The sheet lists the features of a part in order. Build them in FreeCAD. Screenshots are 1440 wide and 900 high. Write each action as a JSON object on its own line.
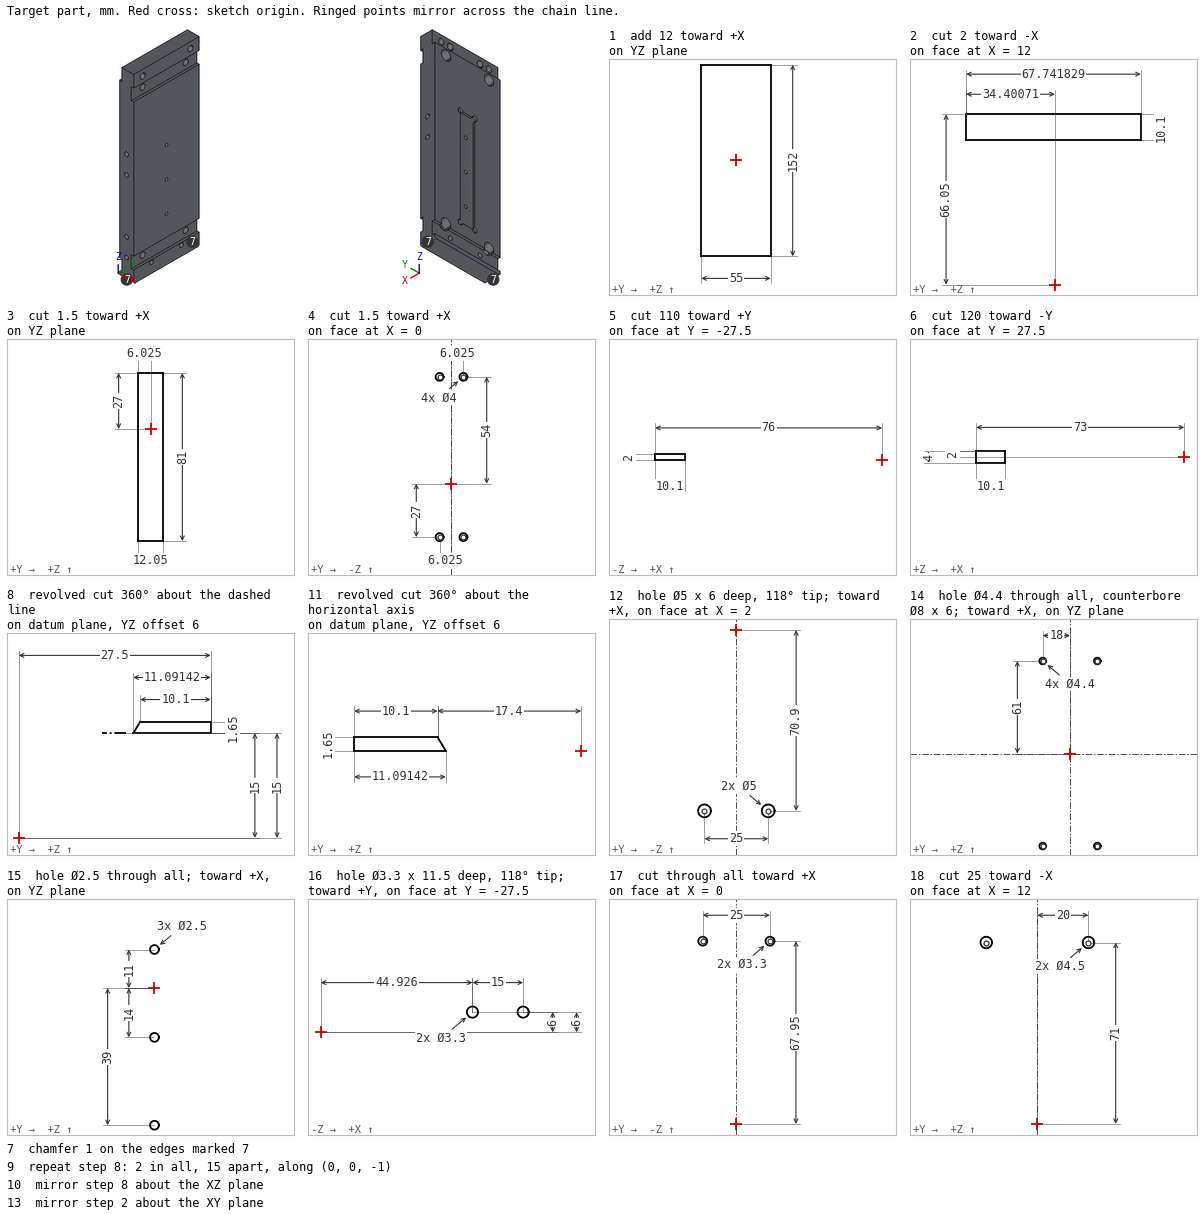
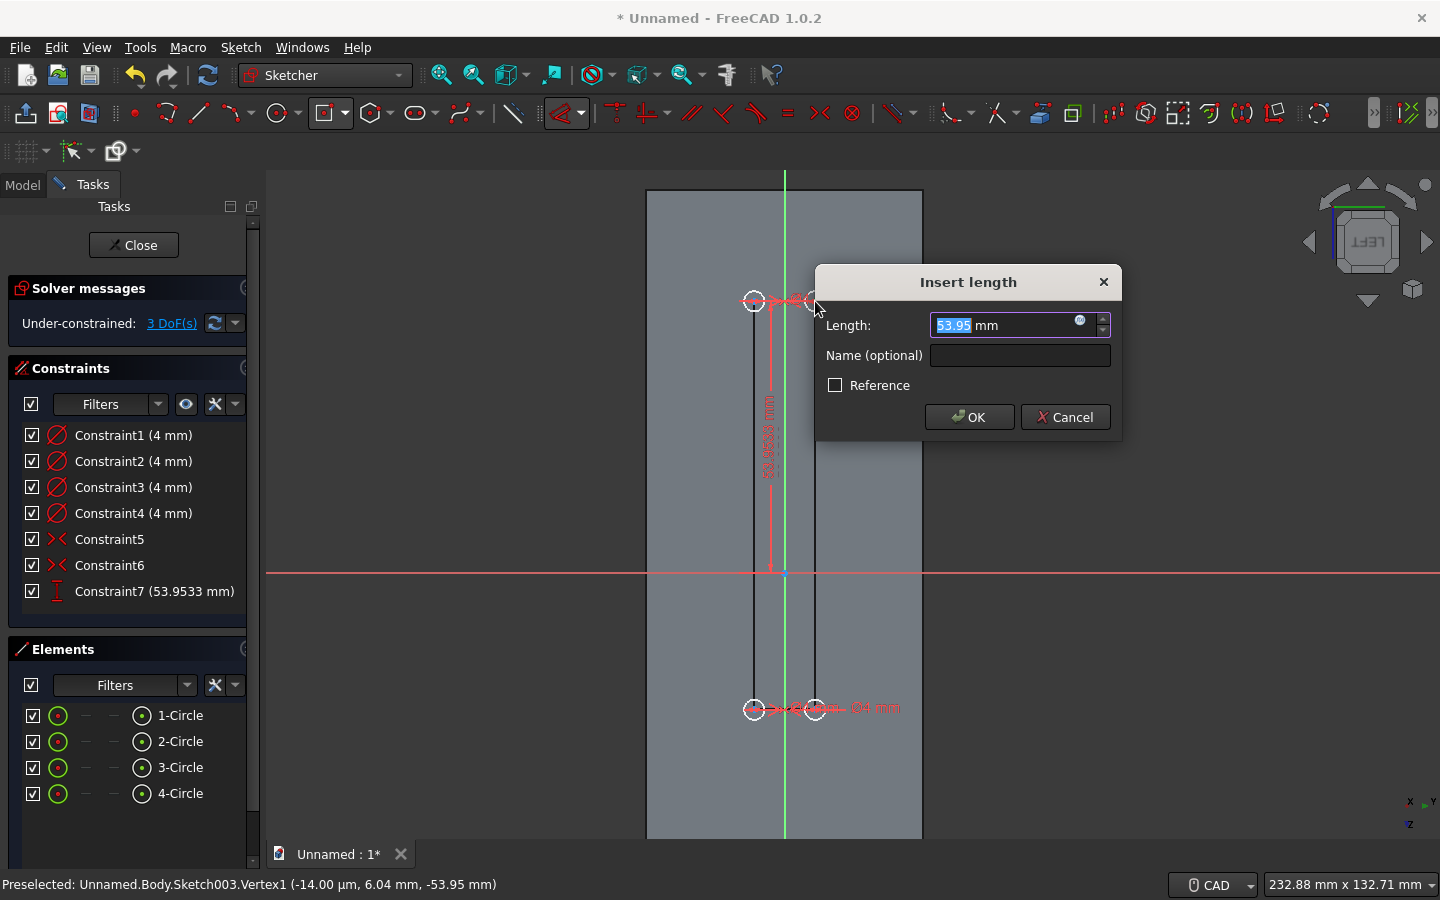
{"action": "type", "text": "54"}
{"action": "key", "text": "Return"}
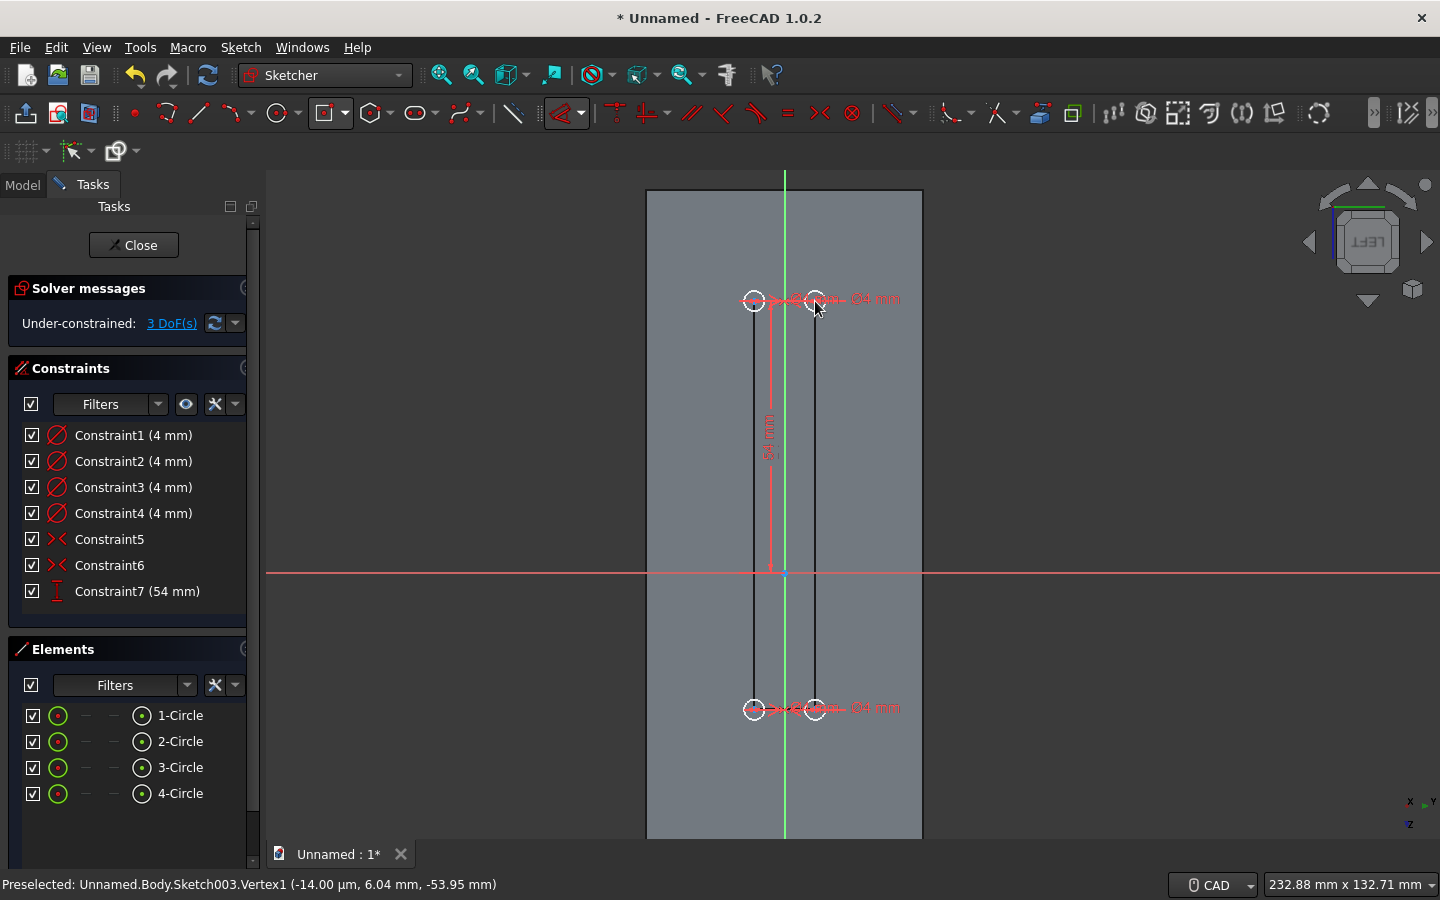
{"action": "left_click", "coordinate": [754, 710]}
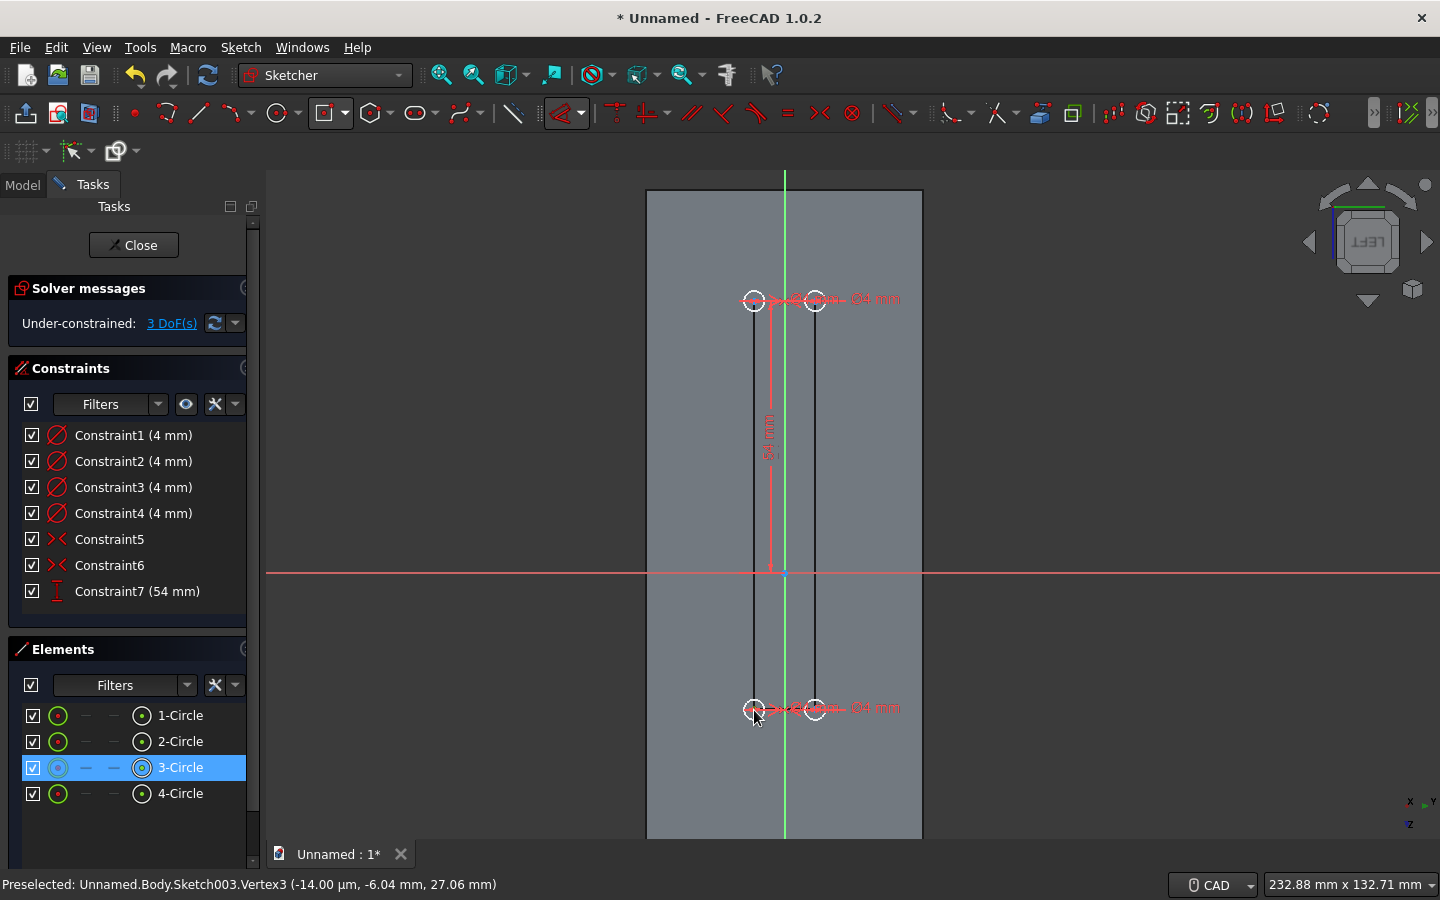
{"action": "left_click", "coordinate": [584, 114]}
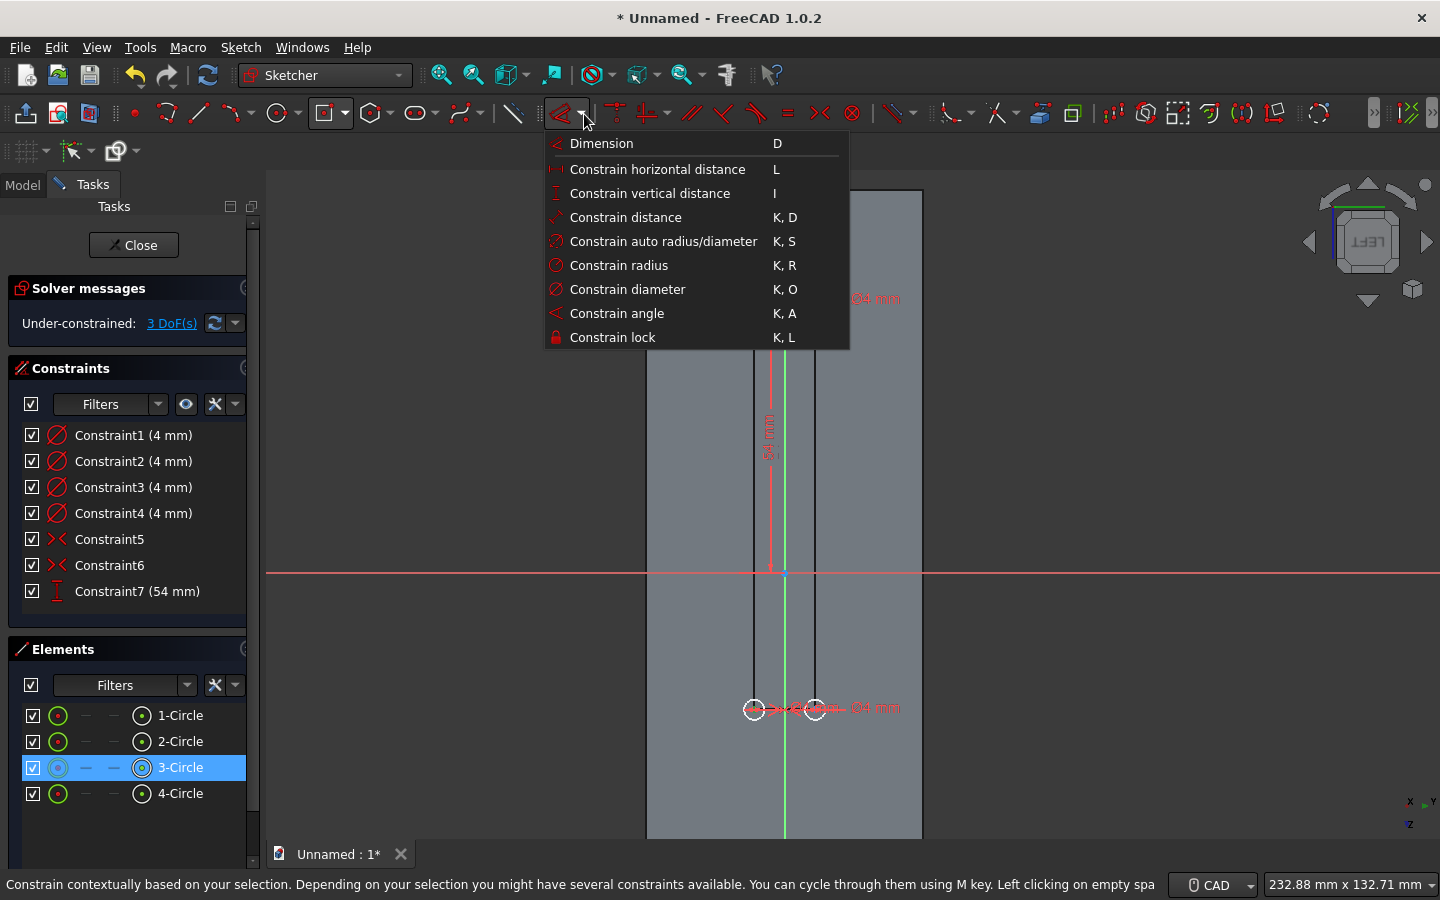
{"action": "left_click", "coordinate": [697, 193]}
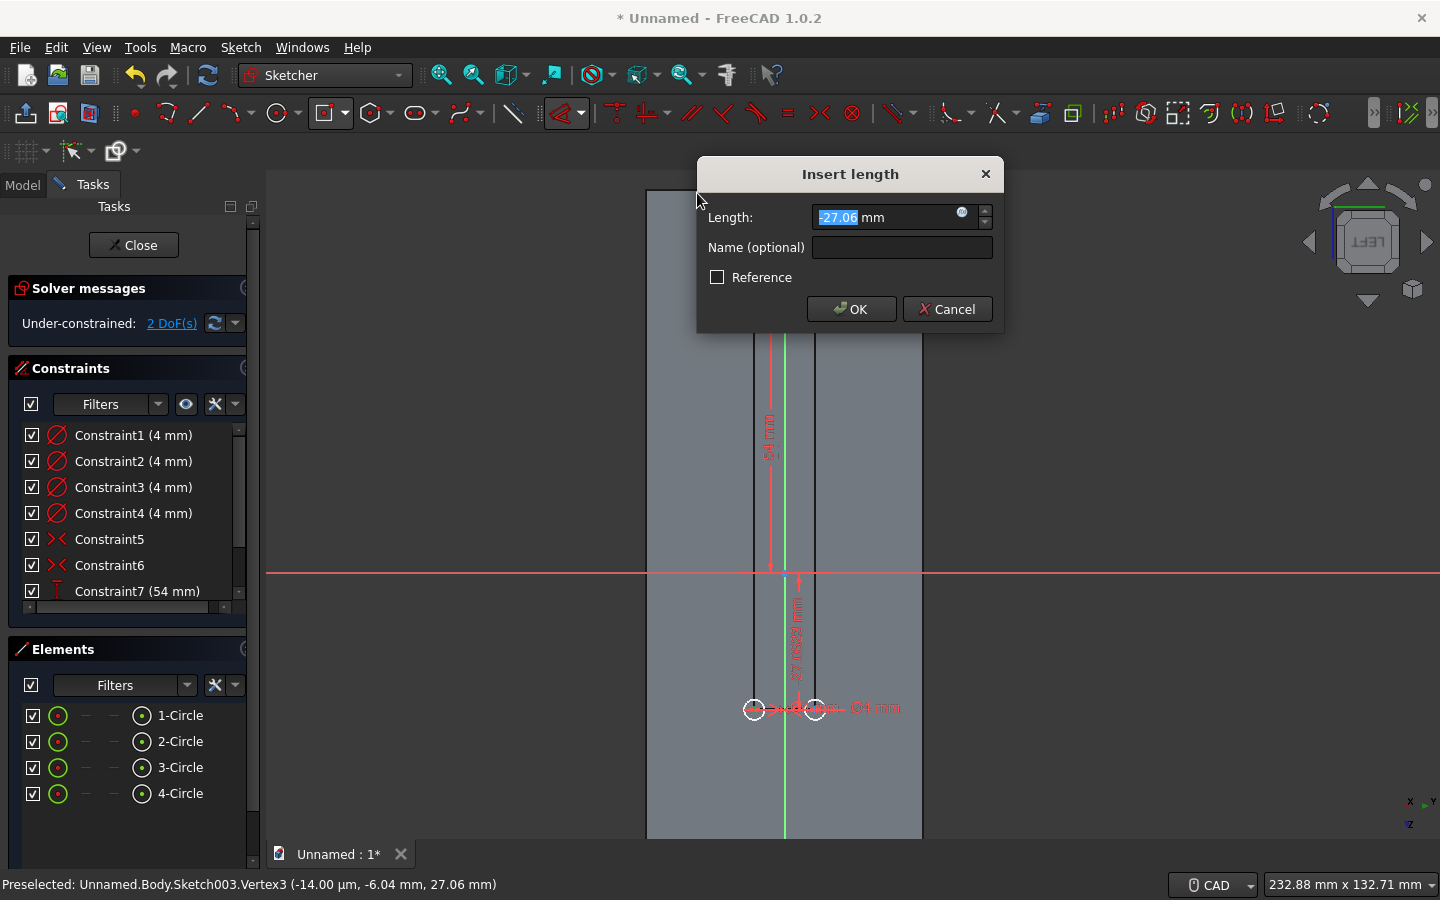
{"action": "type", "text": "-27"}
{"action": "key", "text": "Return"}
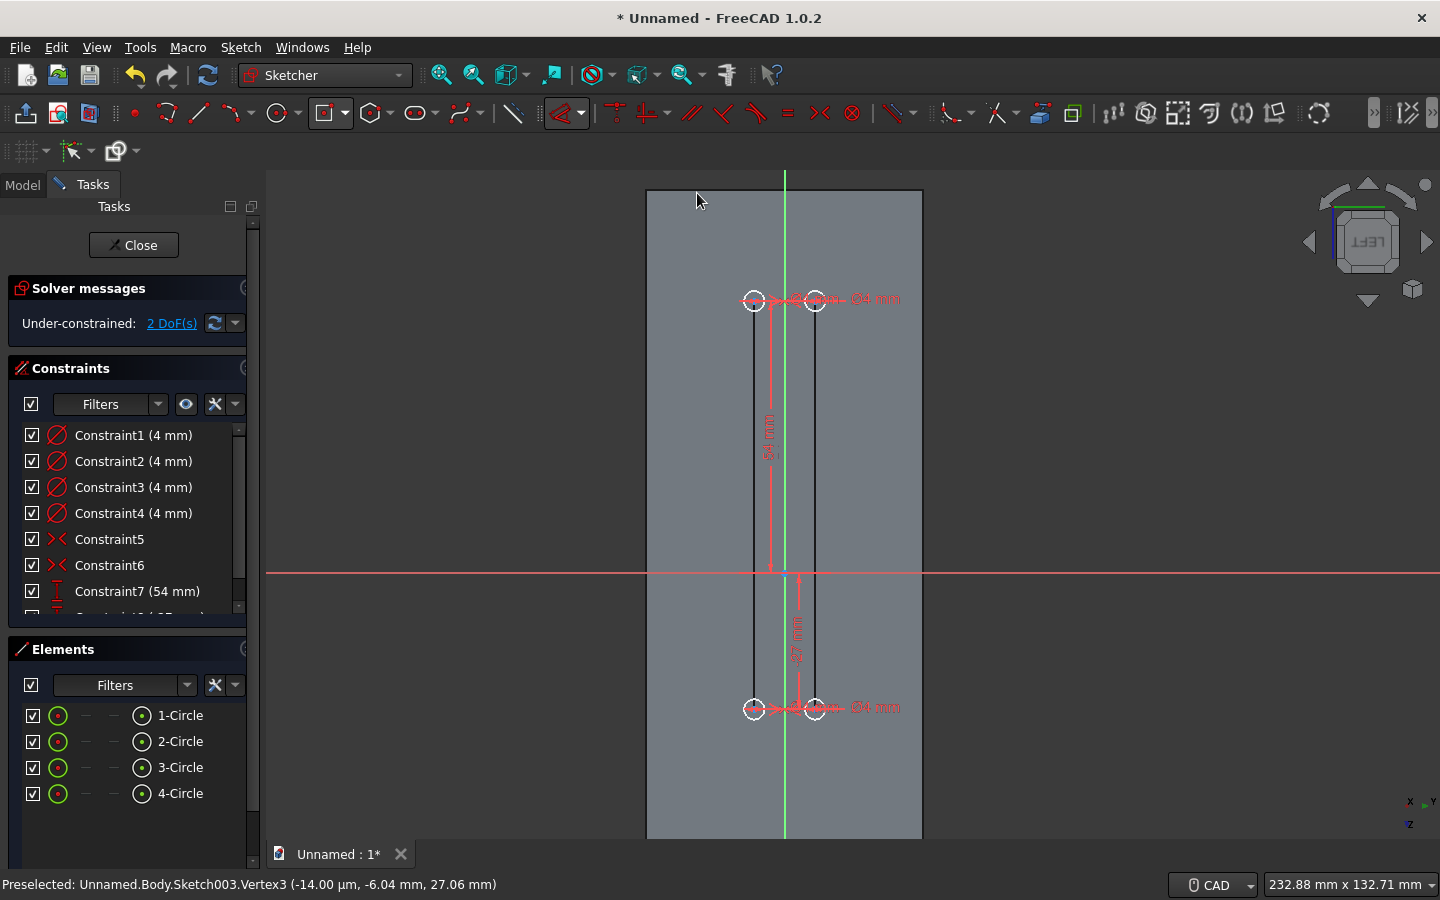
{"action": "scroll", "coordinate": [815, 301], "scroll_direction": "up", "scroll_amount": 2}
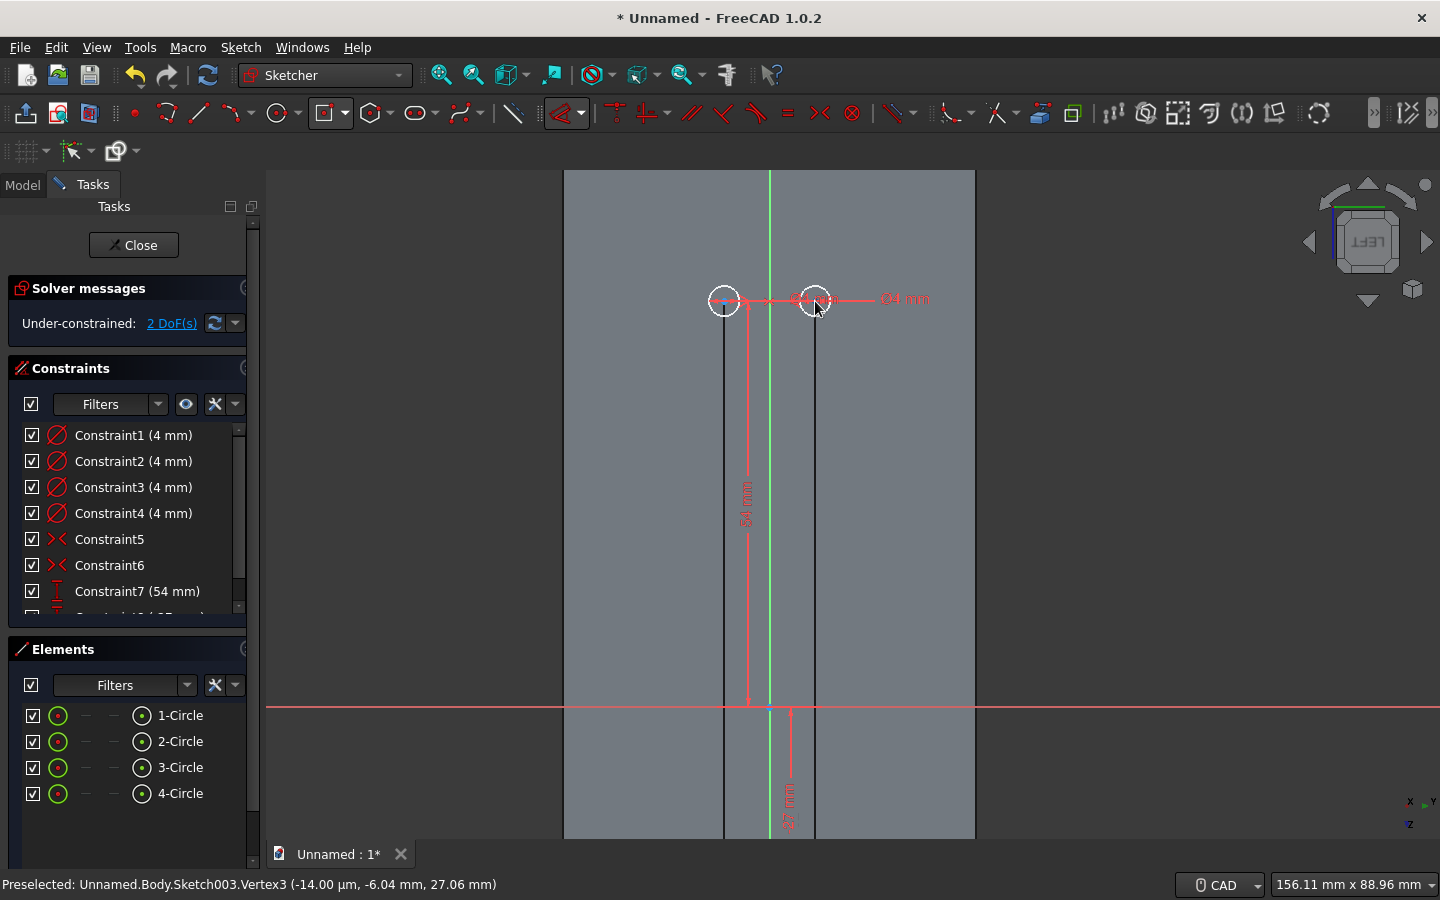
{"action": "left_click", "coordinate": [815, 301]}